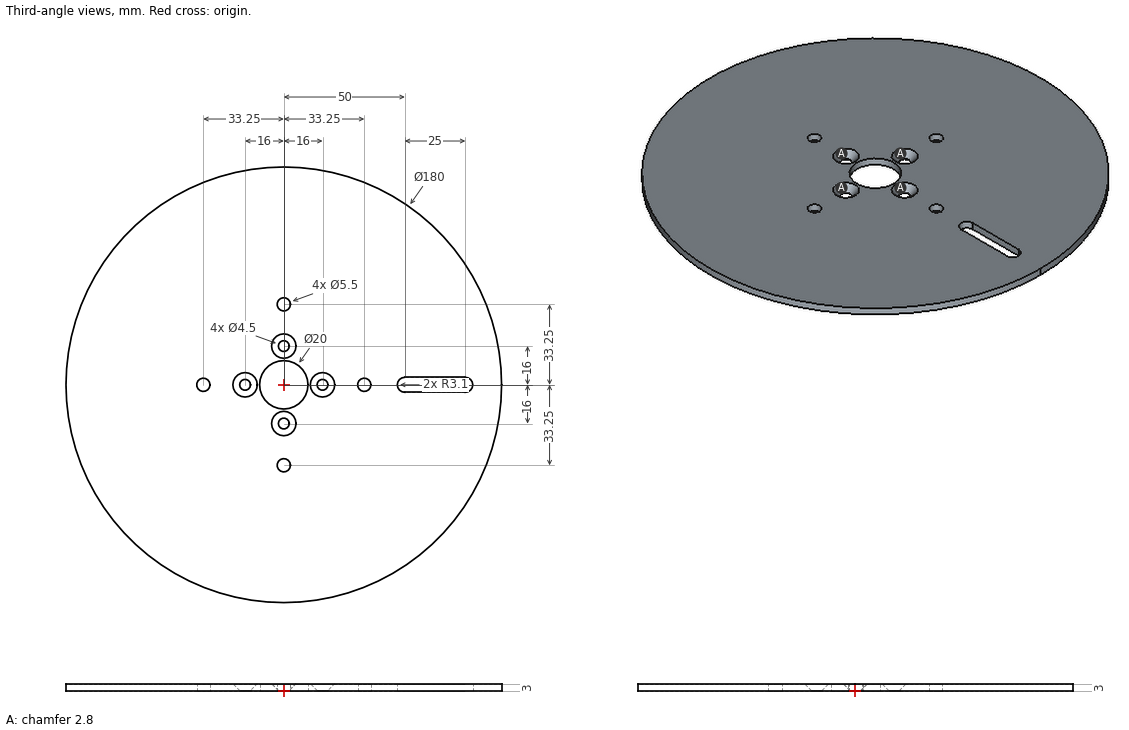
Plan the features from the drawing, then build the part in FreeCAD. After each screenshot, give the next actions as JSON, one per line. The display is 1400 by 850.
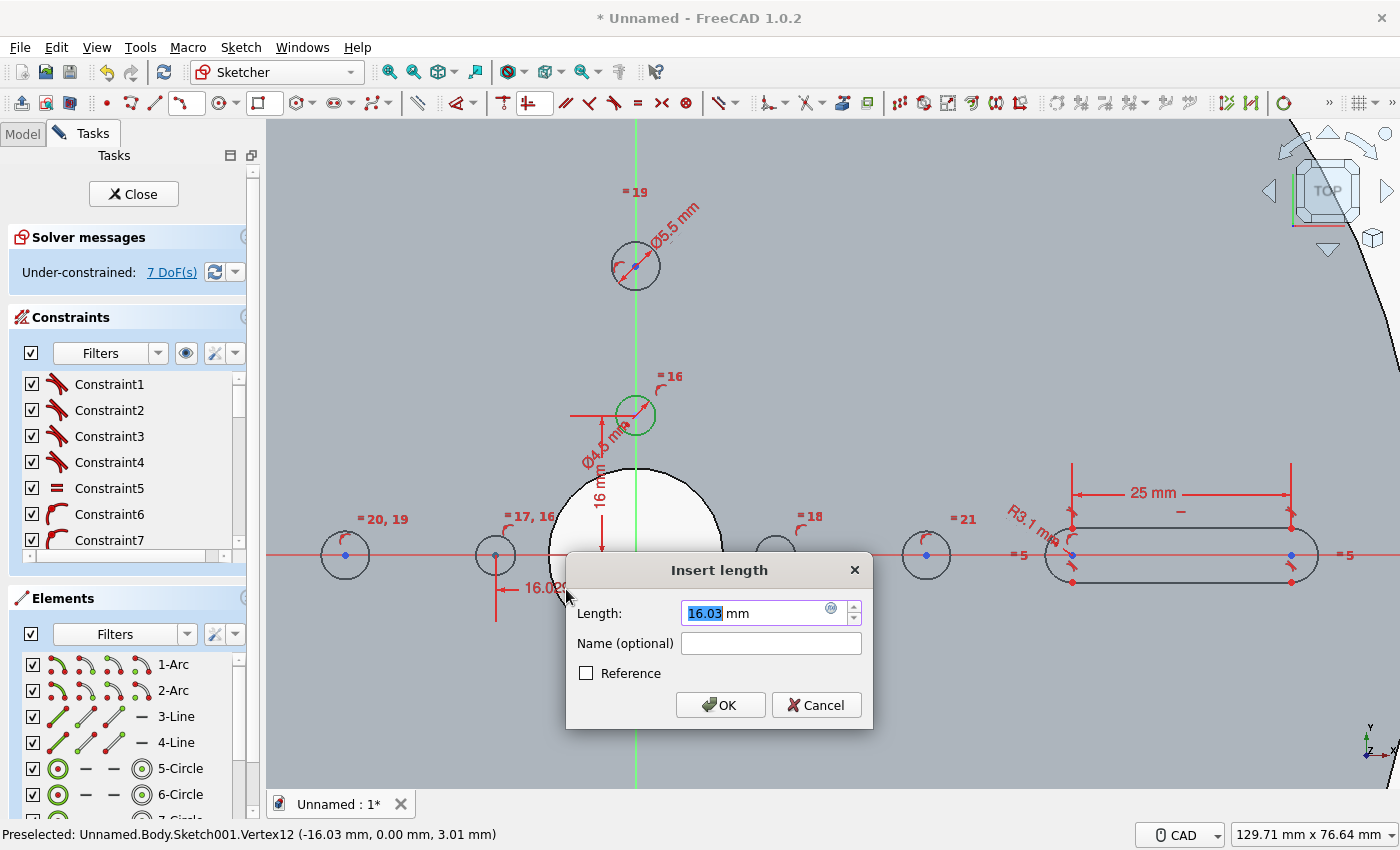
{"action": "type", "text": "16"}
{"action": "key", "text": "Return"}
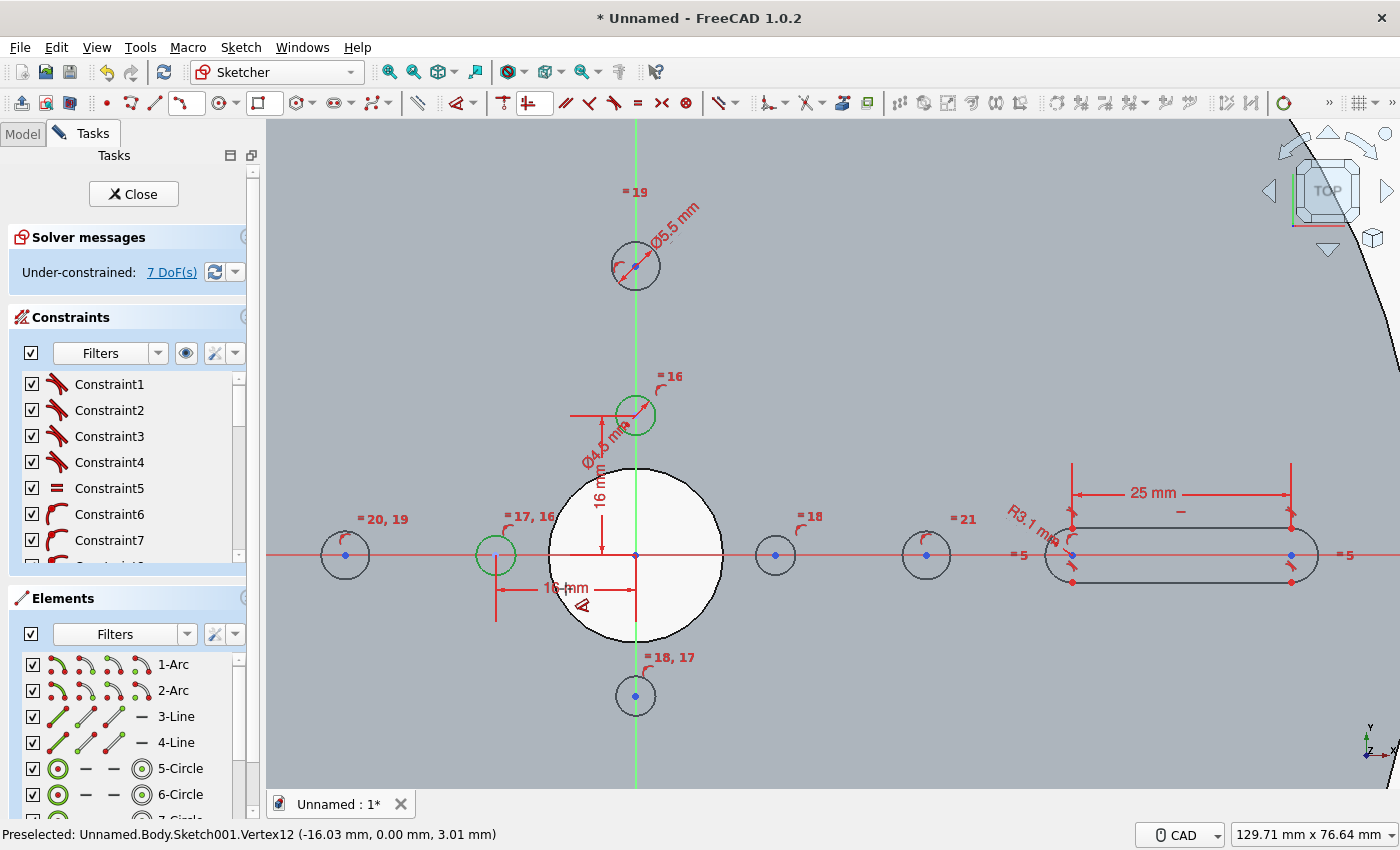
{"action": "left_click", "coordinate": [636, 696]}
{"action": "left_click", "coordinate": [602, 626]}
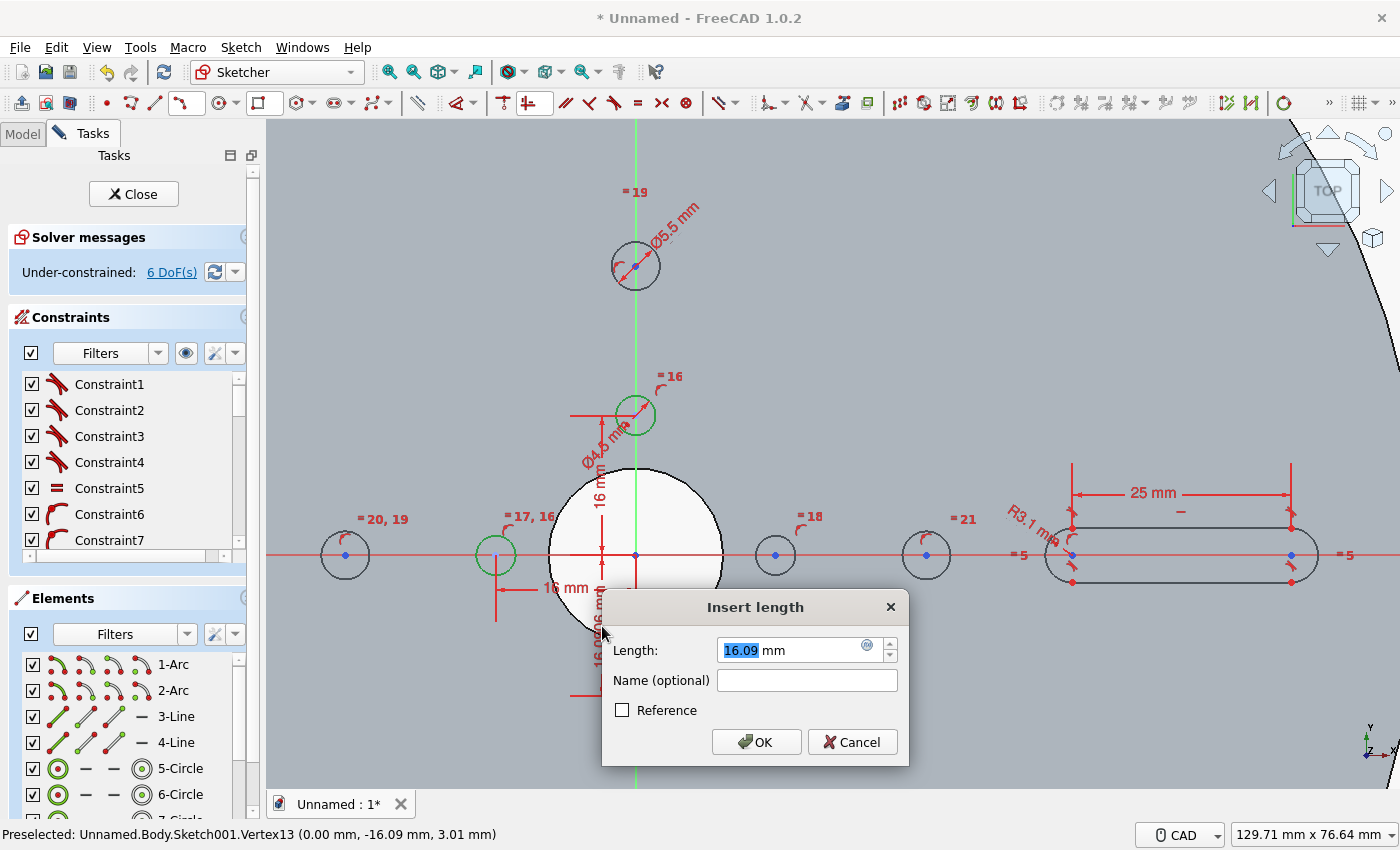
{"action": "type", "text": "16"}
{"action": "key", "text": "Return"}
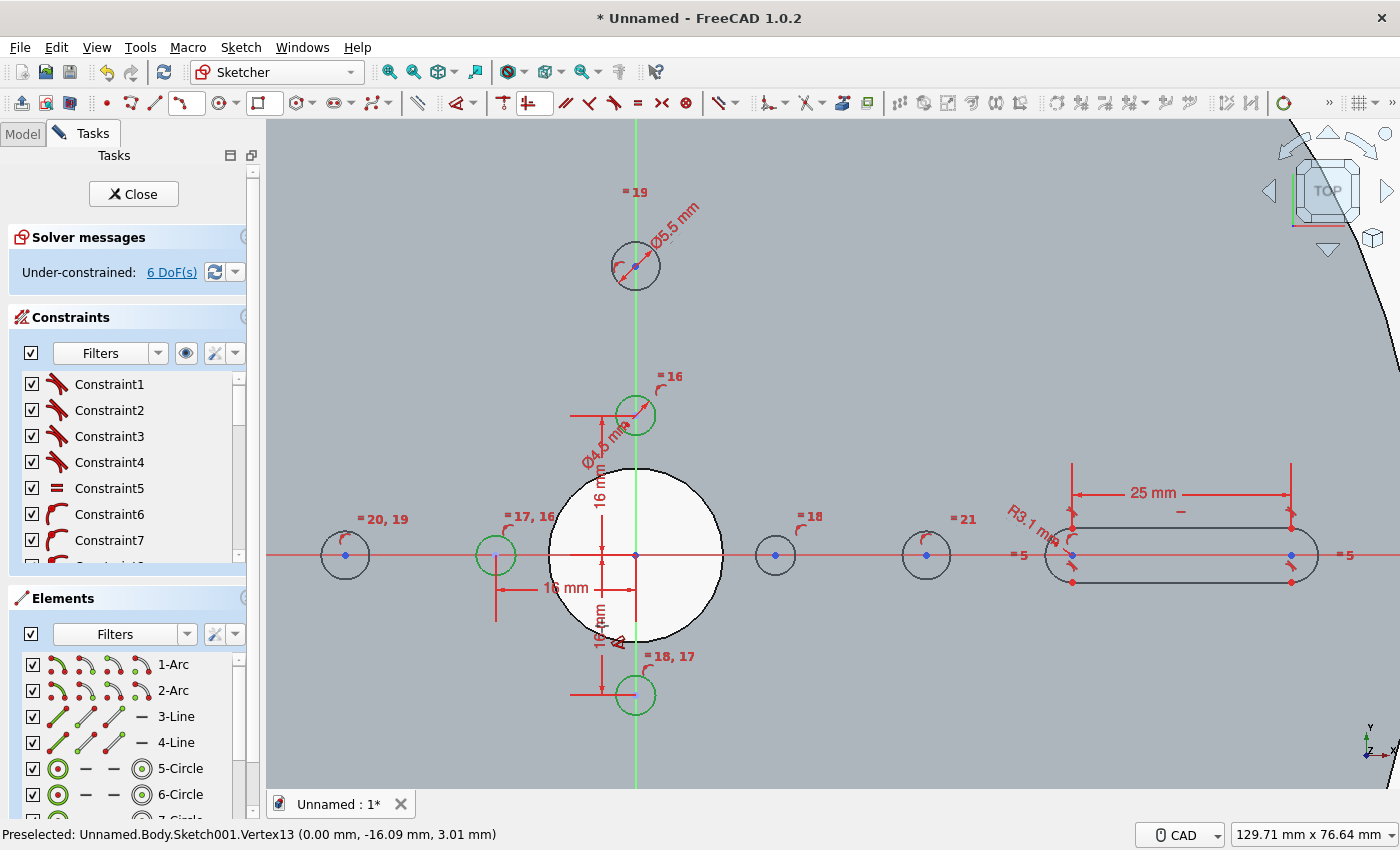
{"action": "left_click", "coordinate": [776, 555]}
{"action": "left_click", "coordinate": [706, 589]}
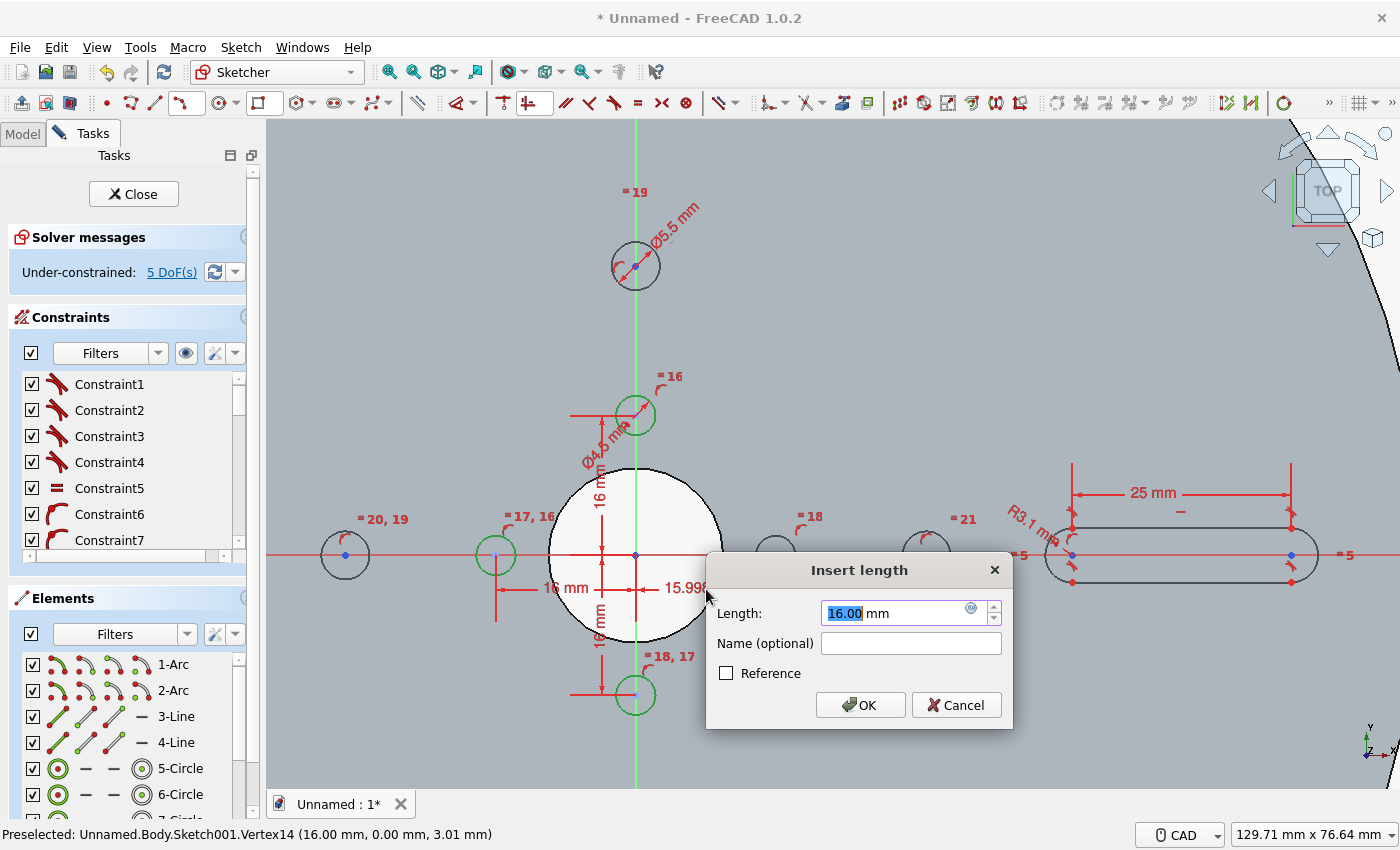
{"action": "type", "text": "16"}
{"action": "key", "text": "Return"}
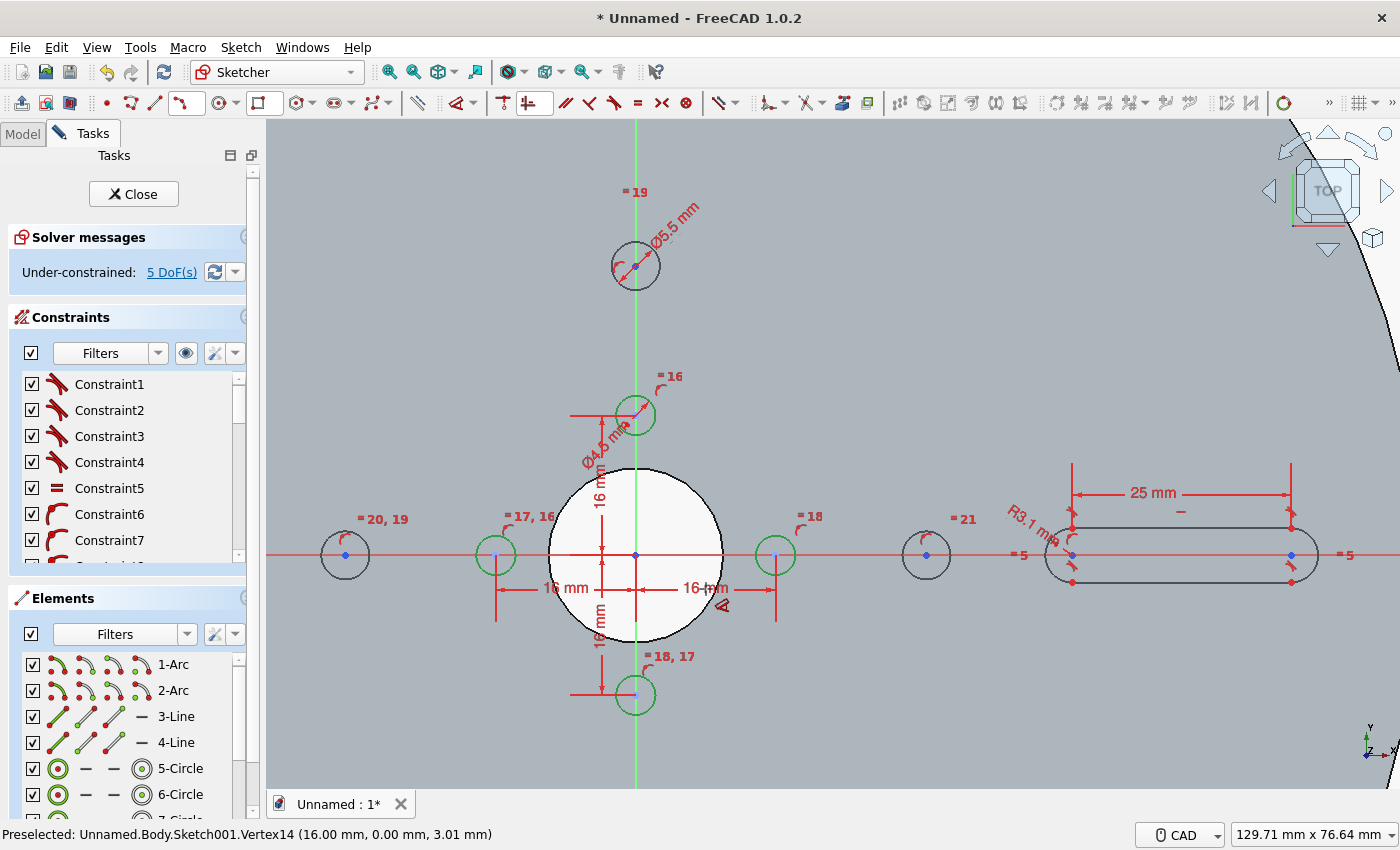
{"action": "left_click", "coordinate": [1072, 528]}
{"action": "left_click", "coordinate": [854, 494]}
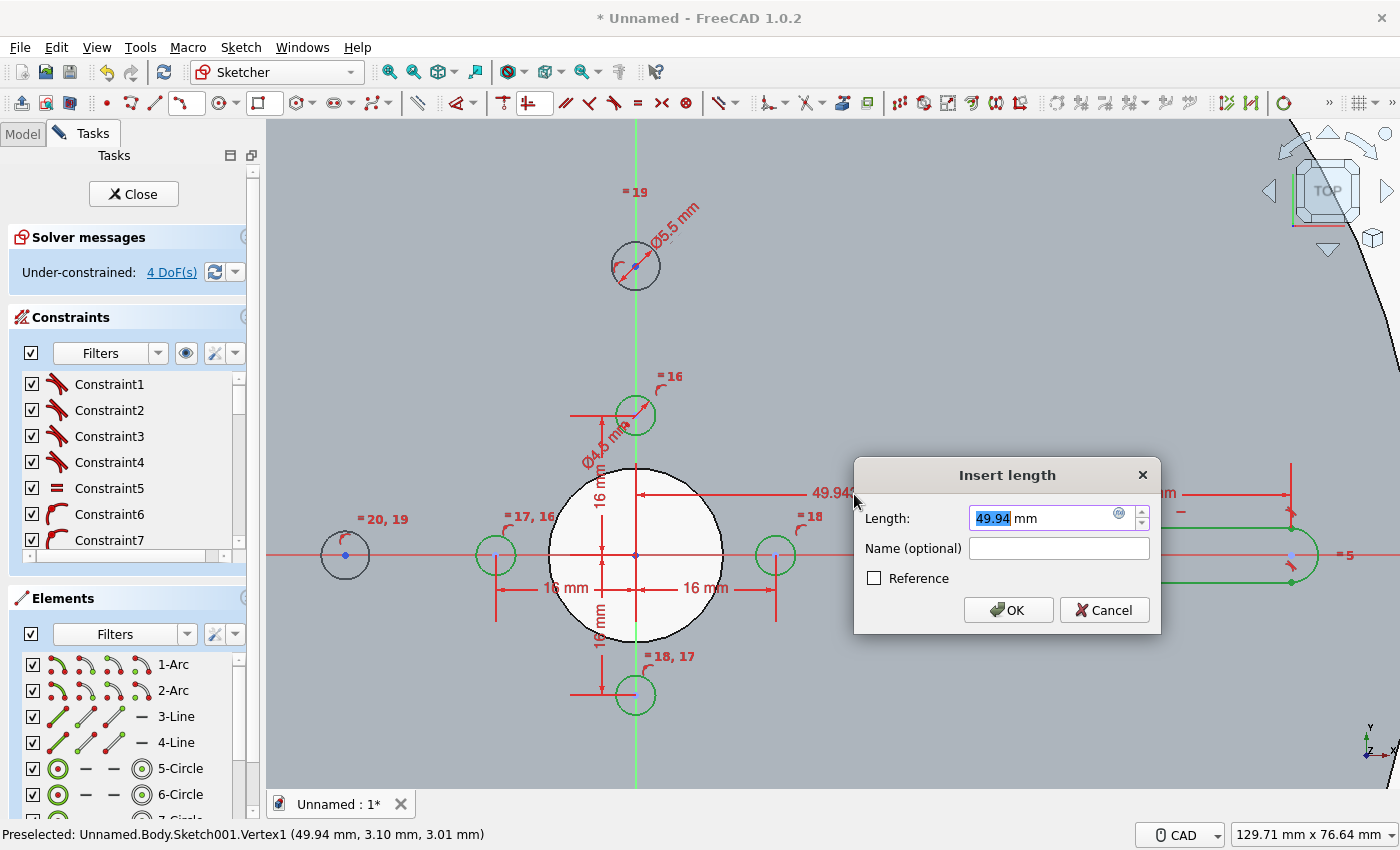
{"action": "type", "text": "50"}
{"action": "key", "text": "Return"}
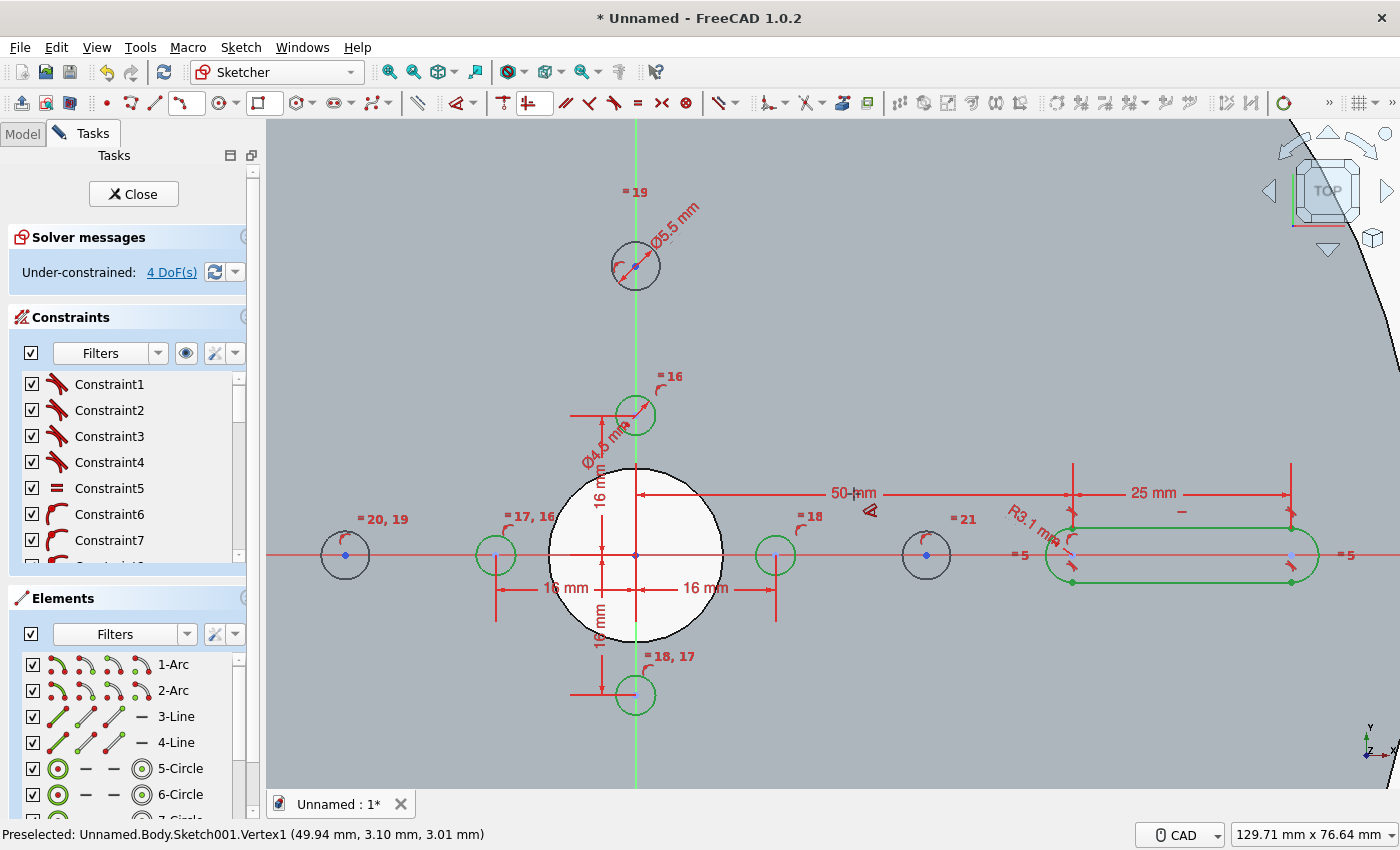
{"action": "left_click", "coordinate": [636, 266]}
{"action": "left_click", "coordinate": [602, 411]}